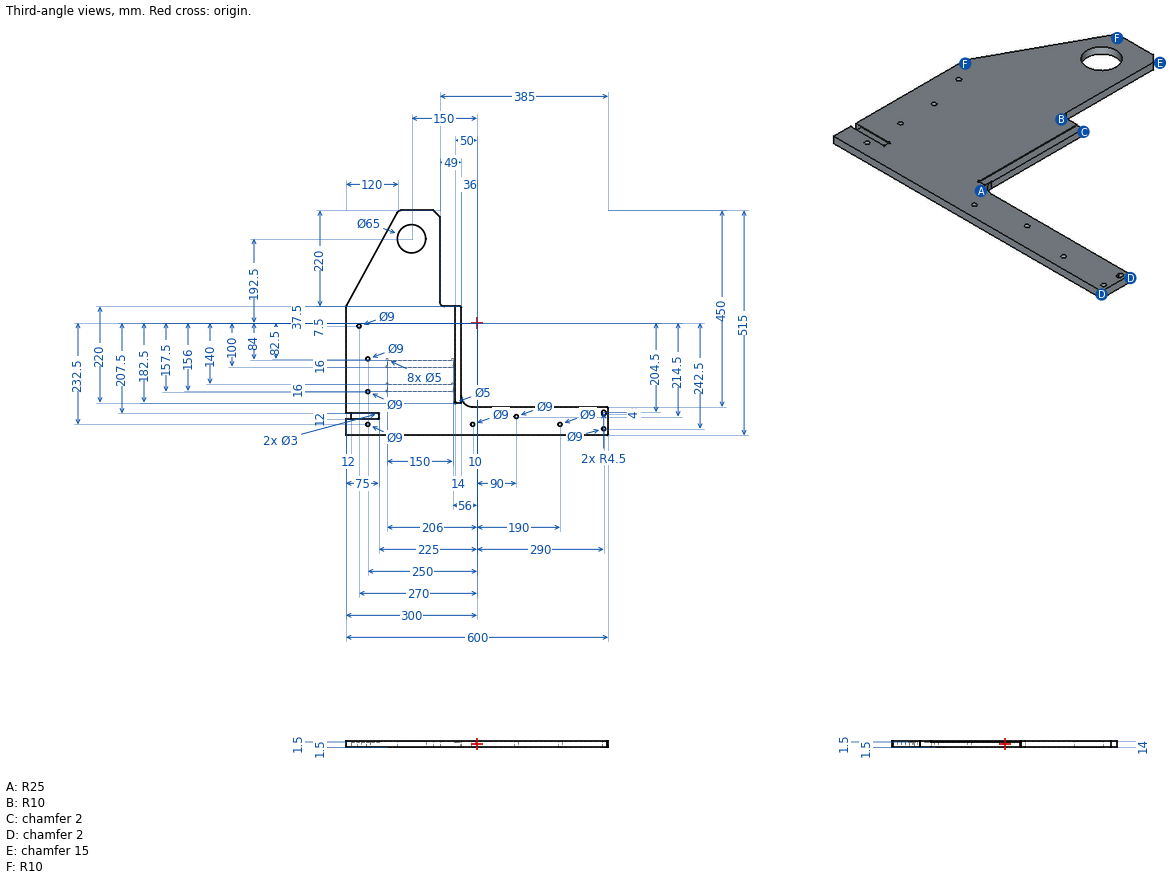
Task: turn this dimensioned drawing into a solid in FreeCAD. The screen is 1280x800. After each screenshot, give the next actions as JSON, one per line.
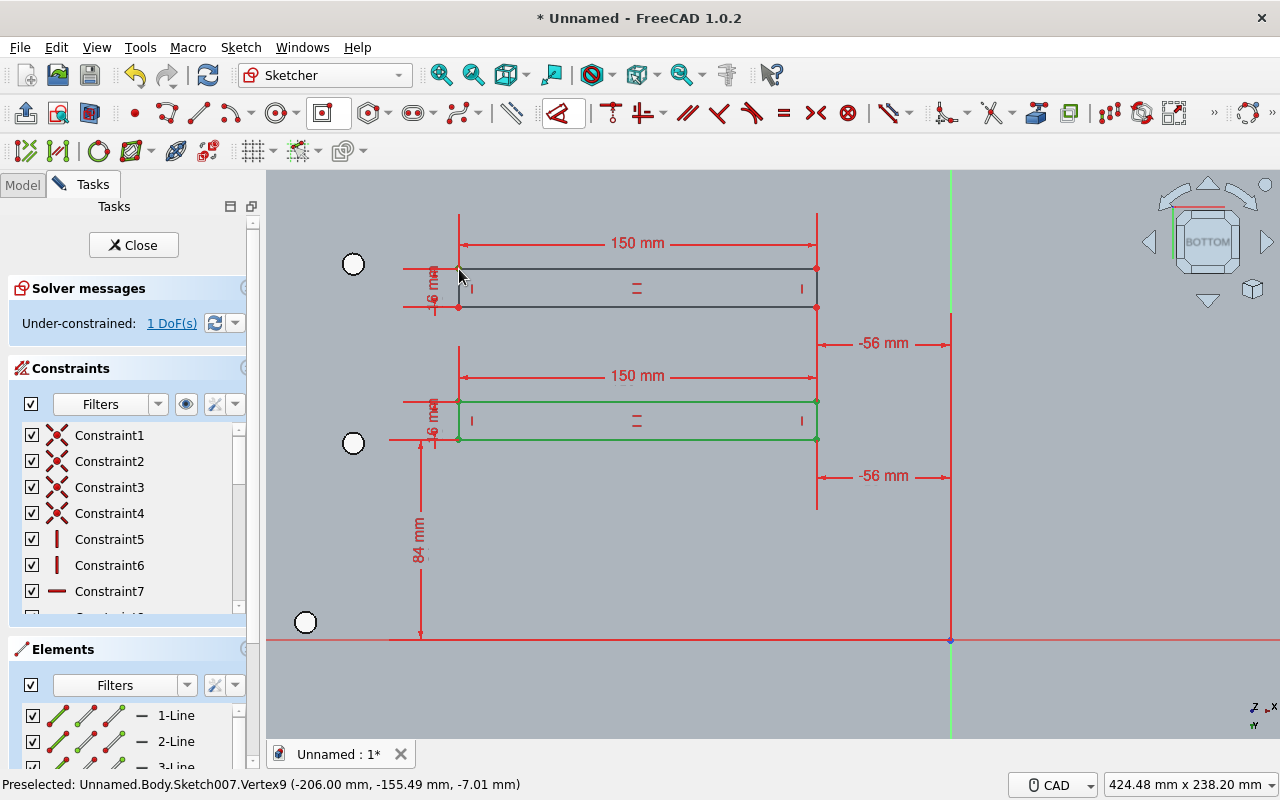
{"action": "left_click", "coordinate": [580, 114]}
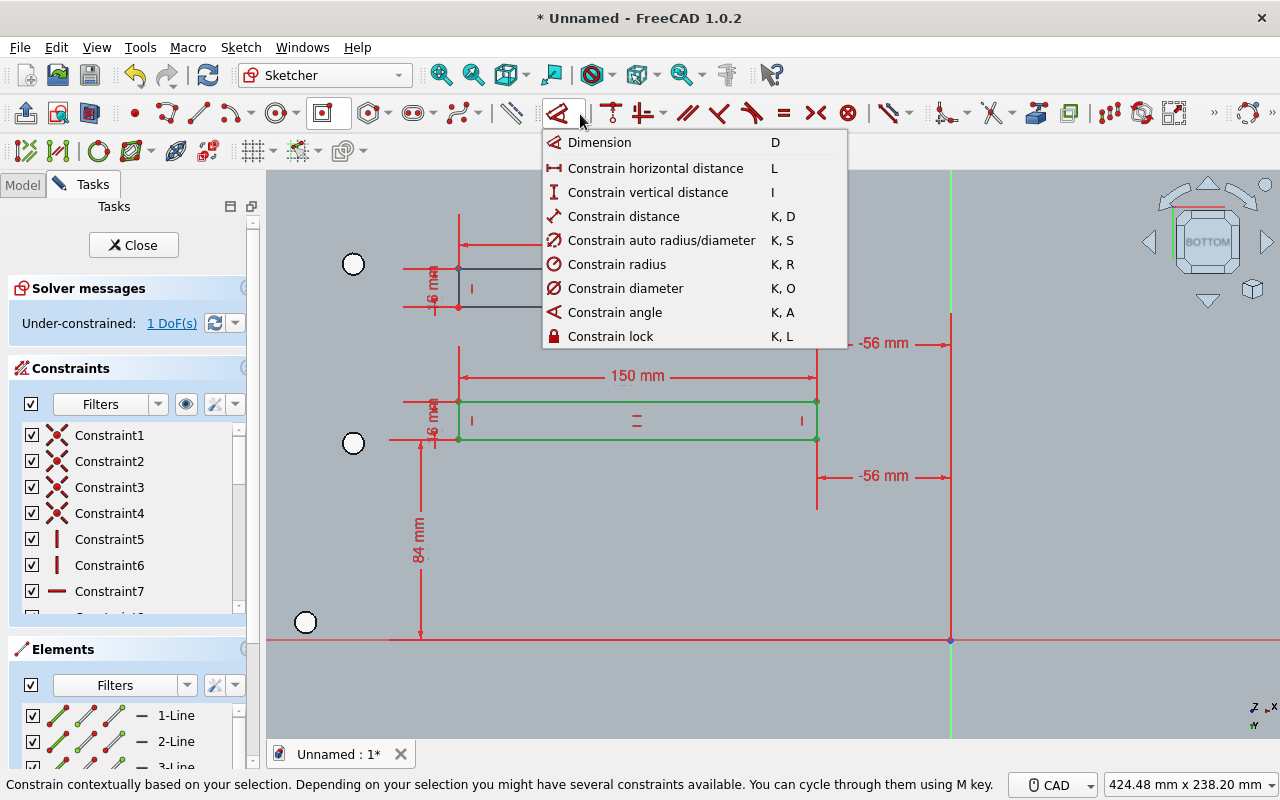
{"action": "left_click", "coordinate": [695, 192]}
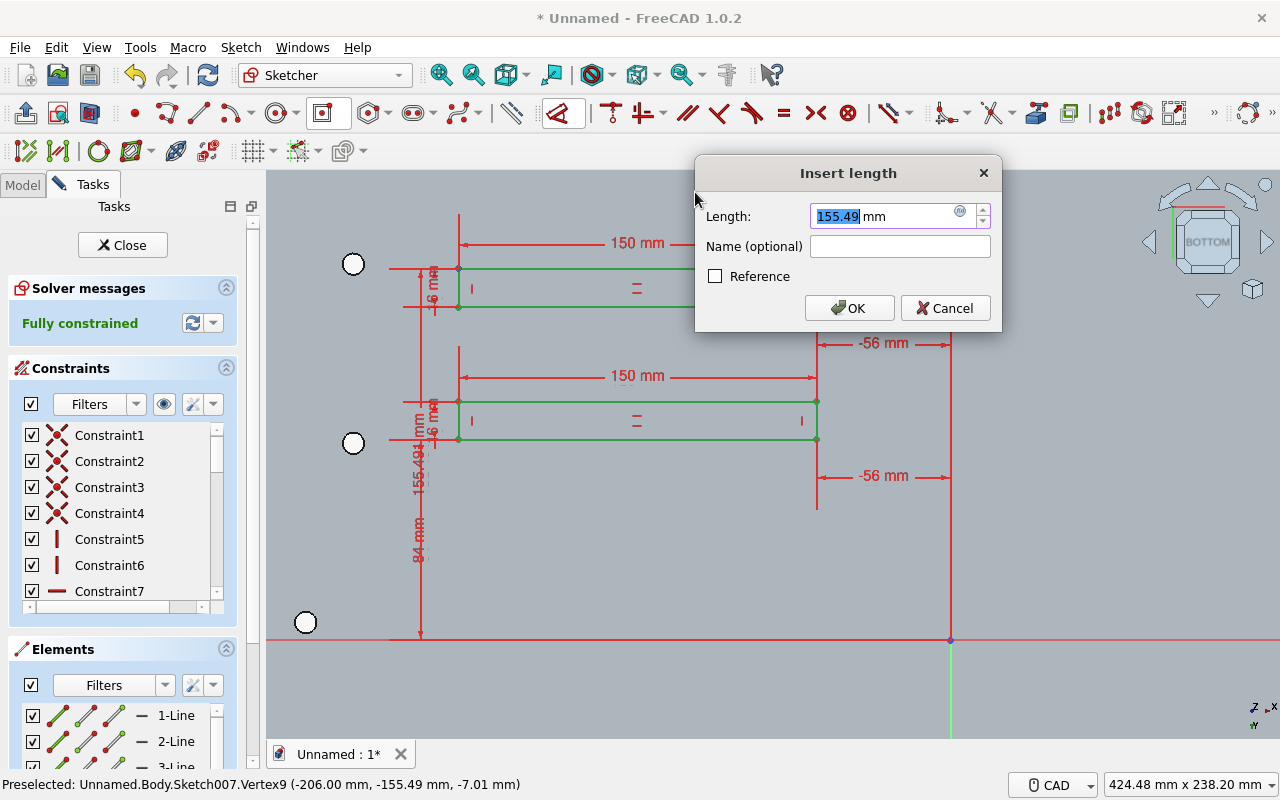
{"action": "type", "text": "156"}
{"action": "key", "text": "Return"}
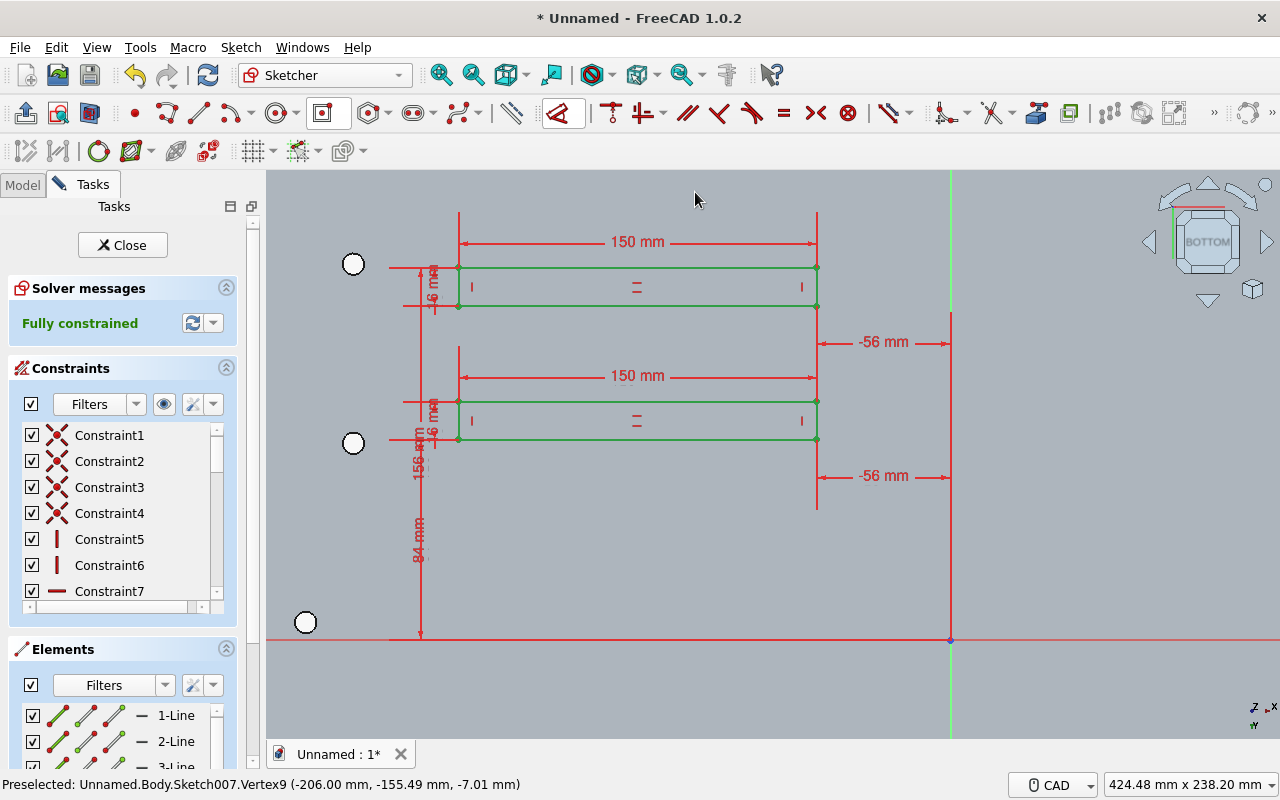
{"action": "left_click", "coordinate": [123, 245]}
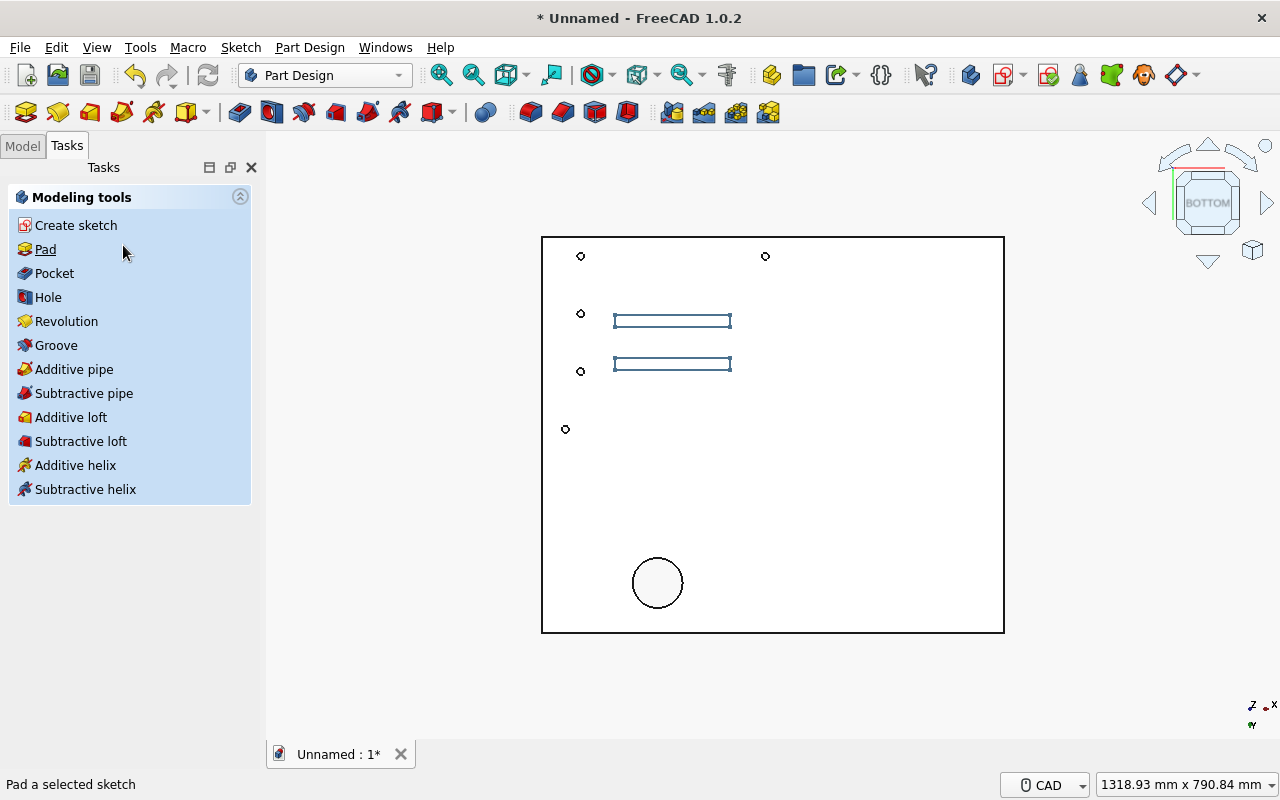
{"action": "left_click", "coordinate": [240, 112]}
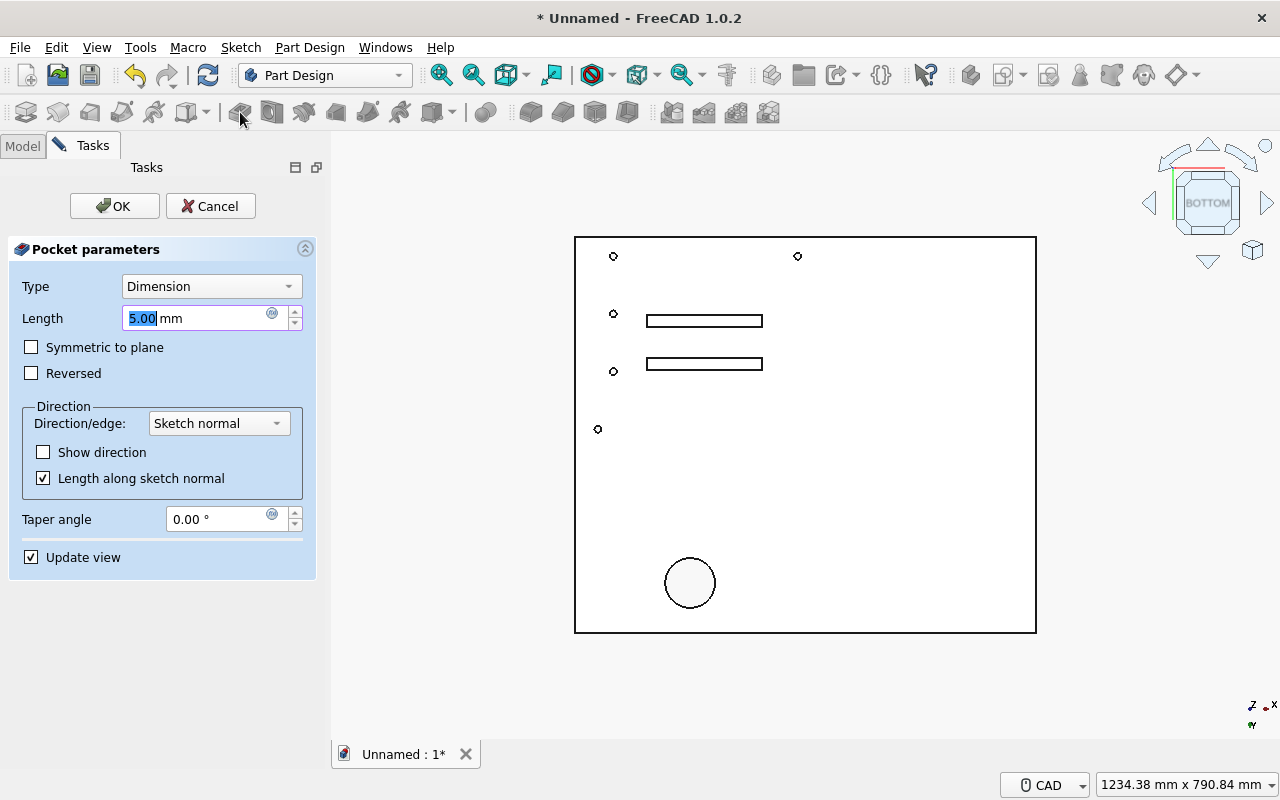
{"action": "type", "text": "1.5"}
{"action": "key", "text": "Tab"}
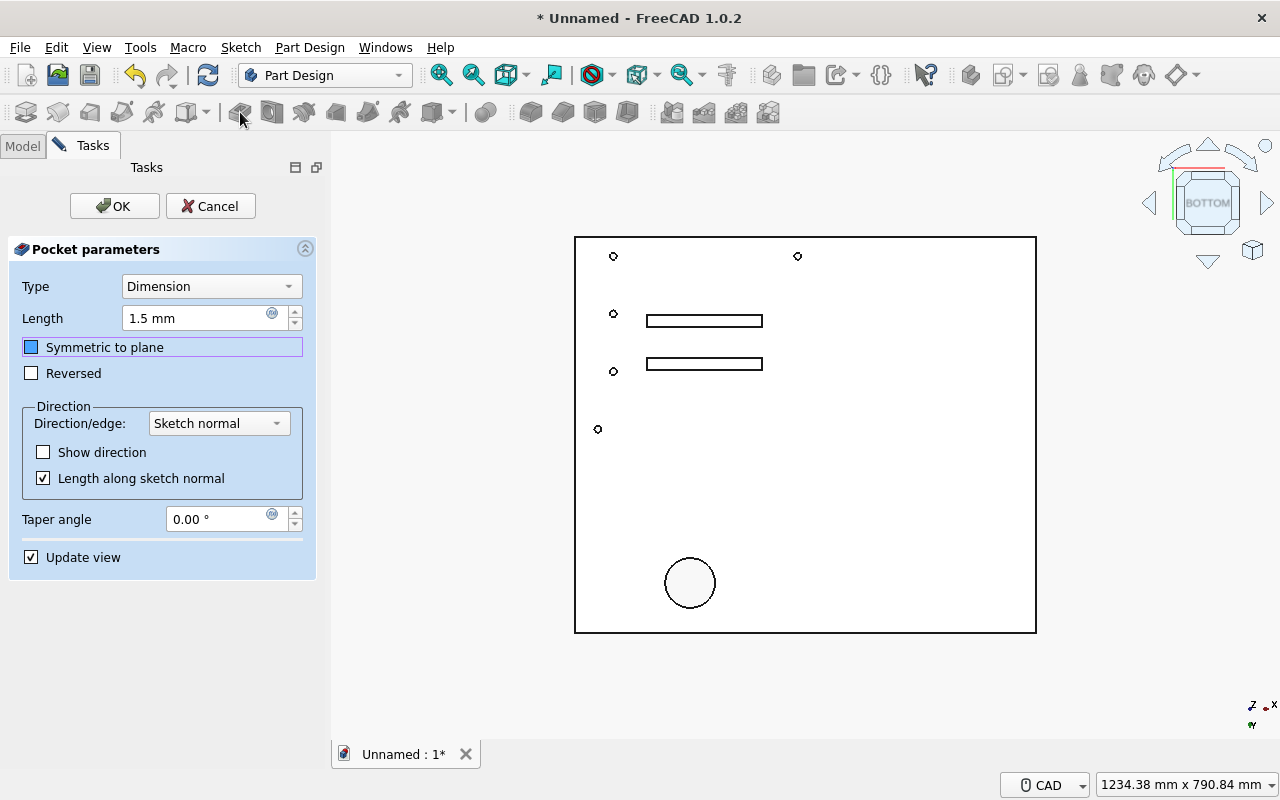
{"action": "left_click", "coordinate": [115, 206]}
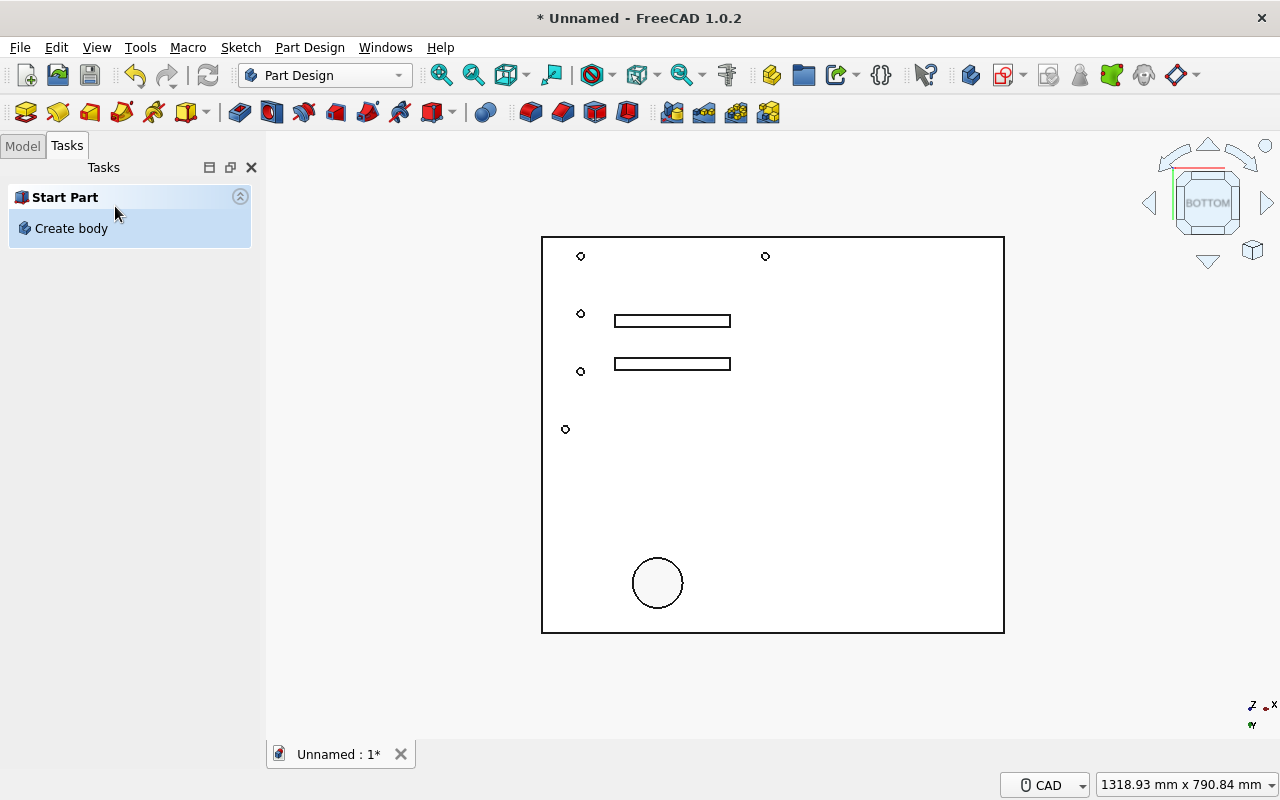
{"action": "left_click", "coordinate": [839, 491]}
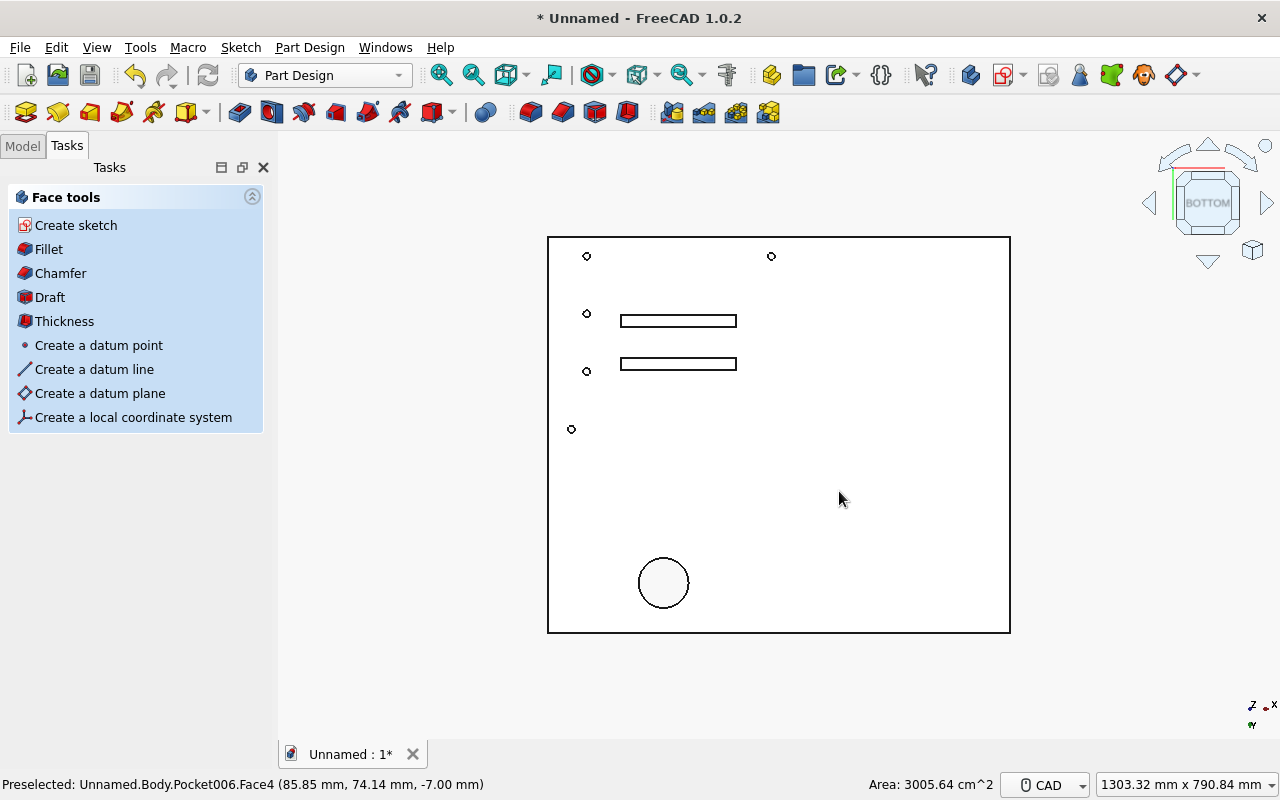
{"action": "left_click", "coordinate": [1004, 76]}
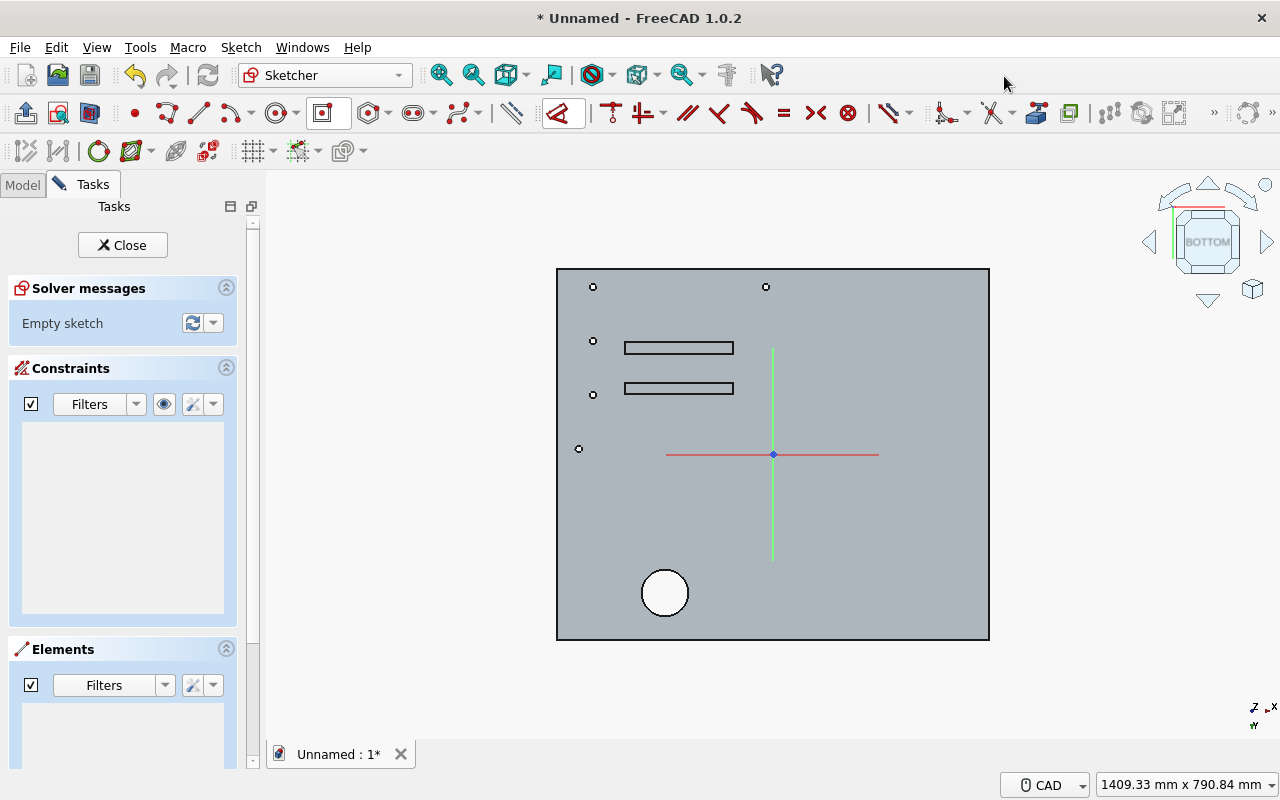
{"action": "scroll", "coordinate": [695, 373], "scroll_direction": "up", "scroll_amount": 6}